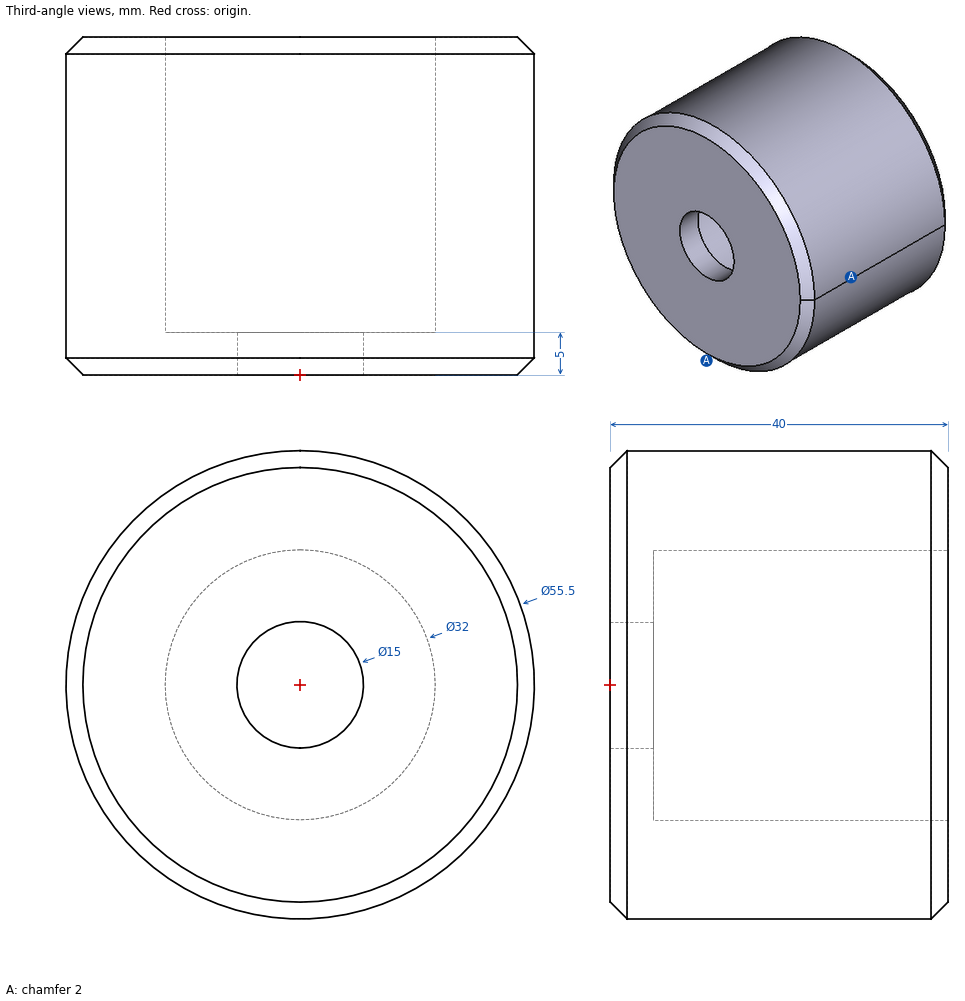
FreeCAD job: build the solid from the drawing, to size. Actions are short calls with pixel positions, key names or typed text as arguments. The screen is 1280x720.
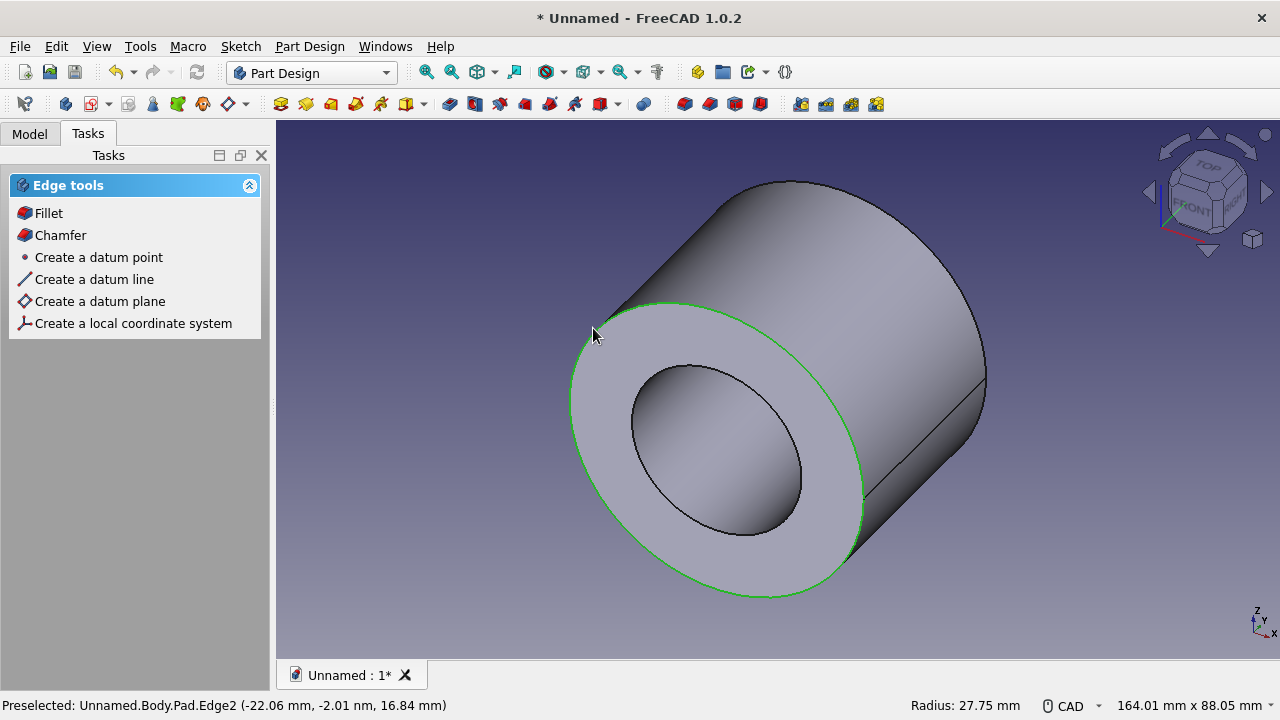
key(0)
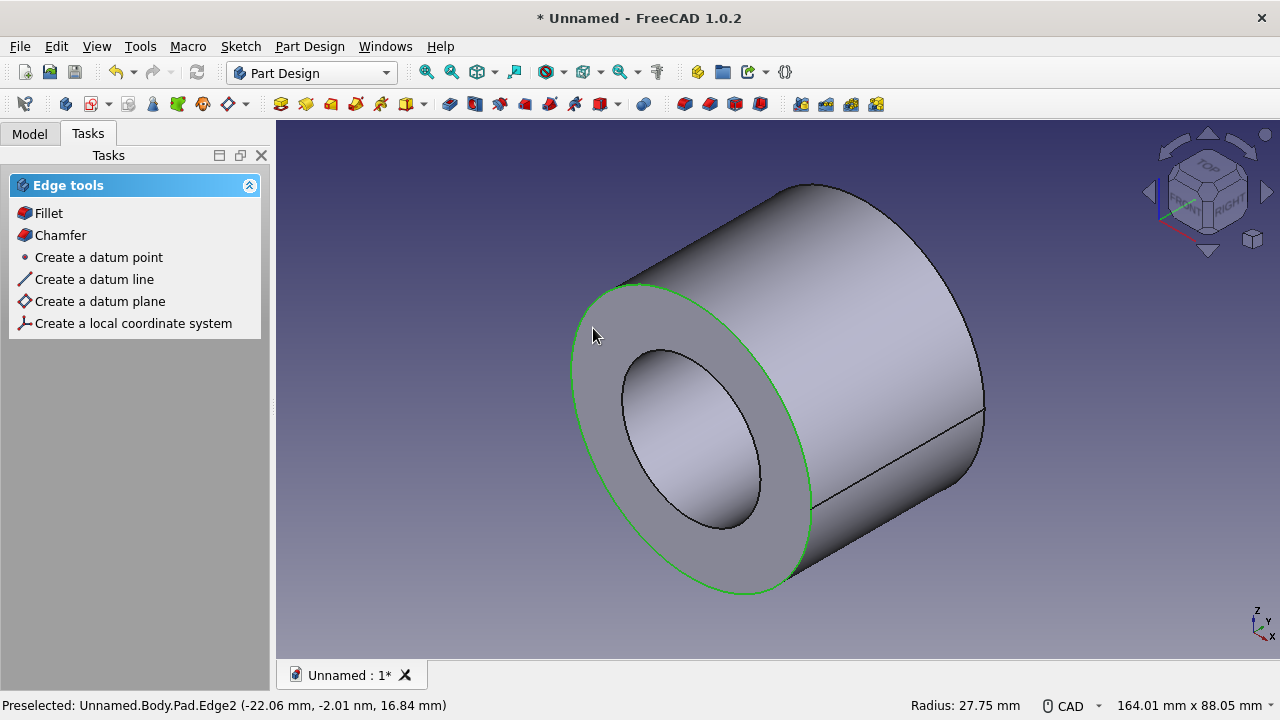
key(2)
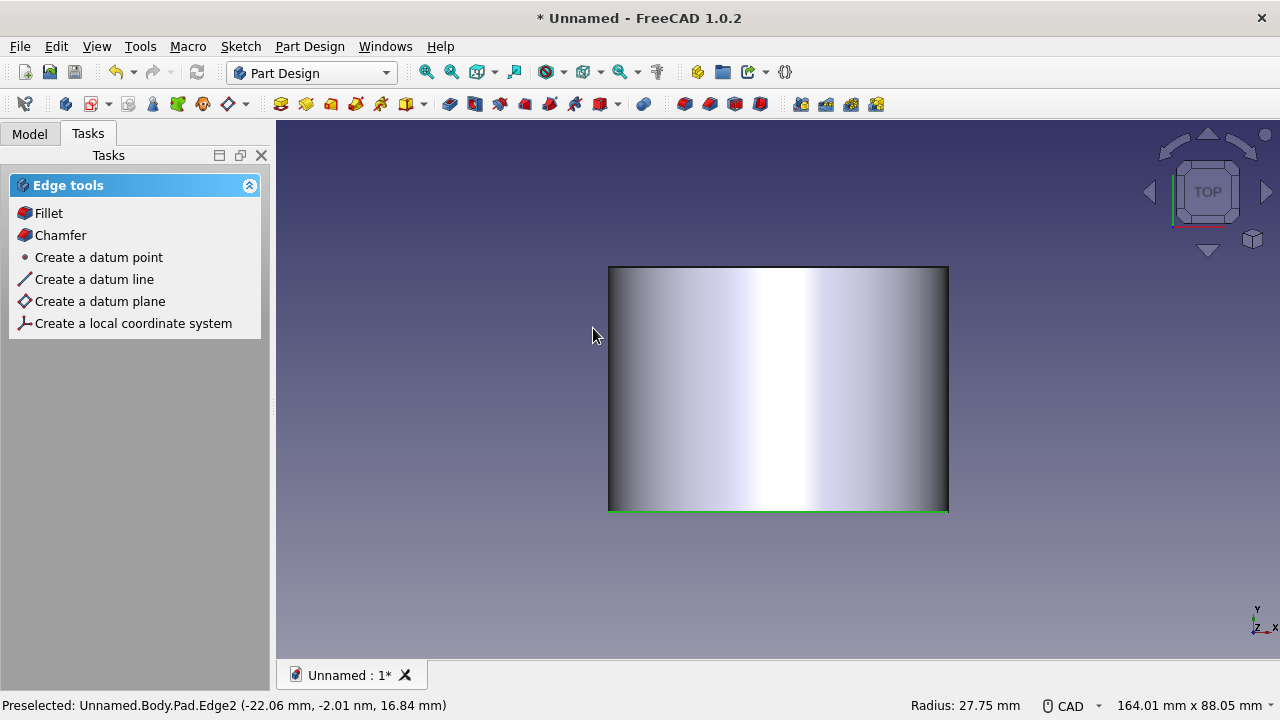
click(640, 266, ctrl)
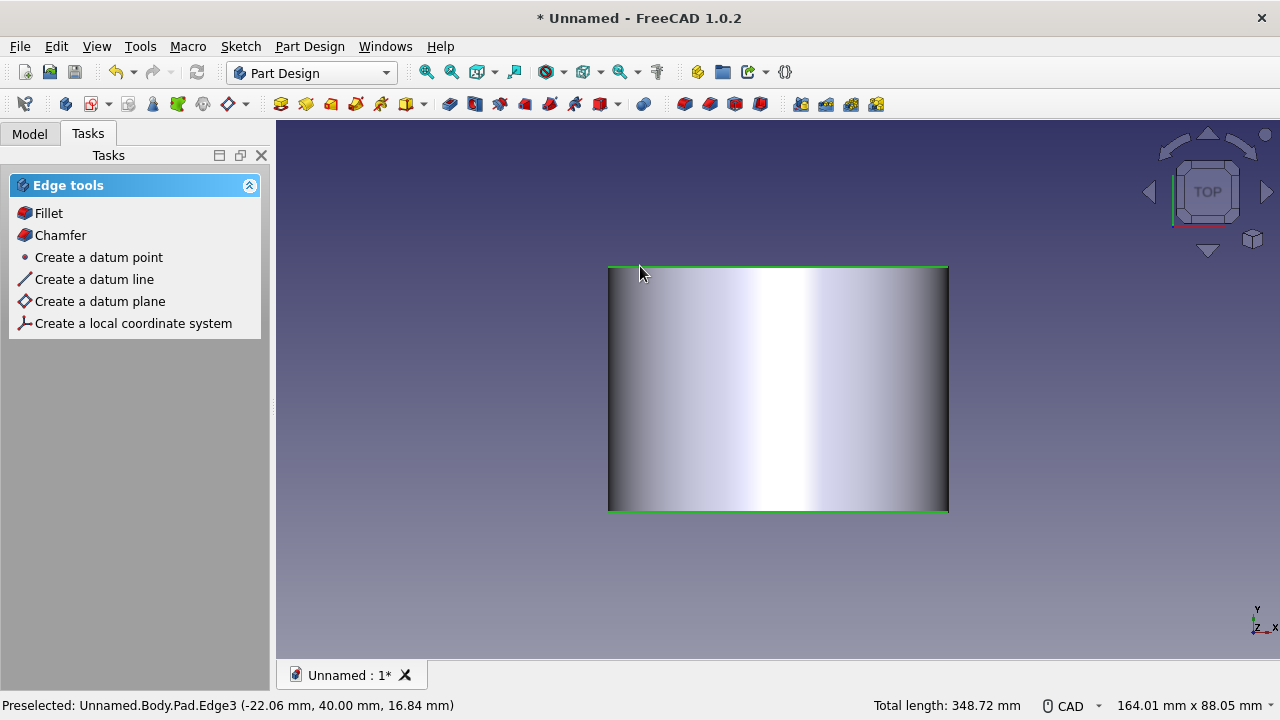
click(710, 104)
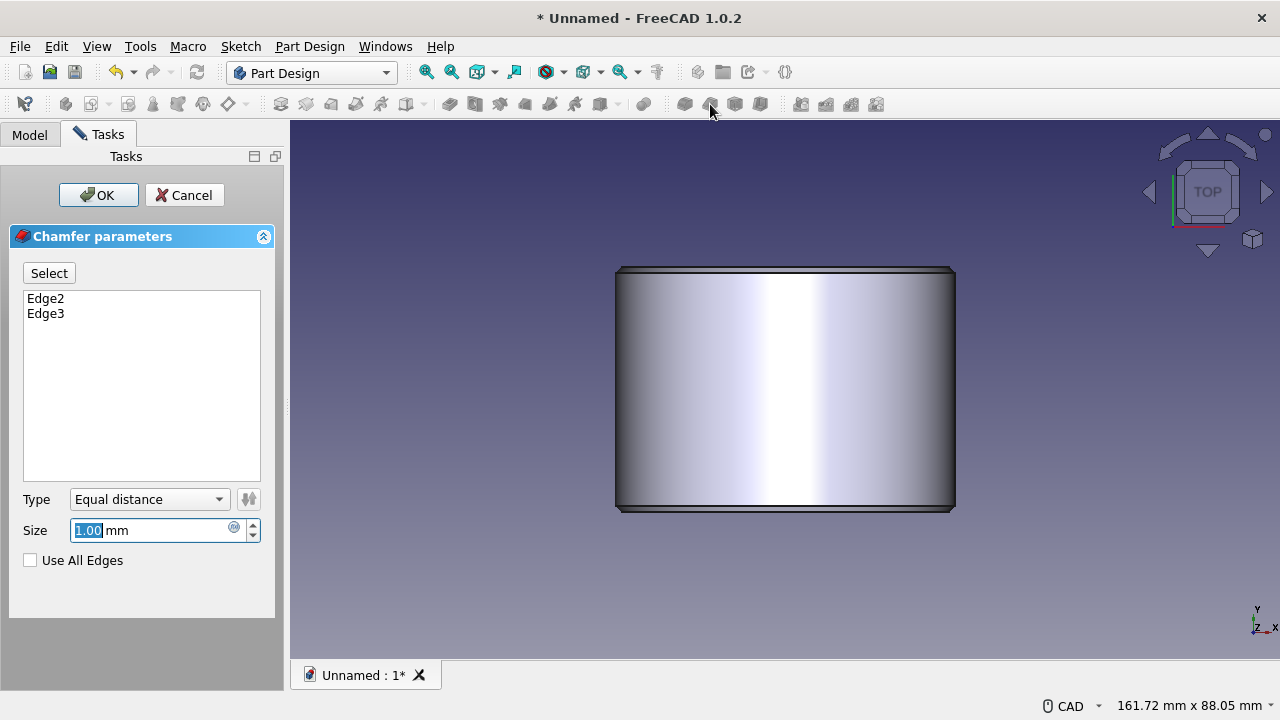
text(2)
key(Tab)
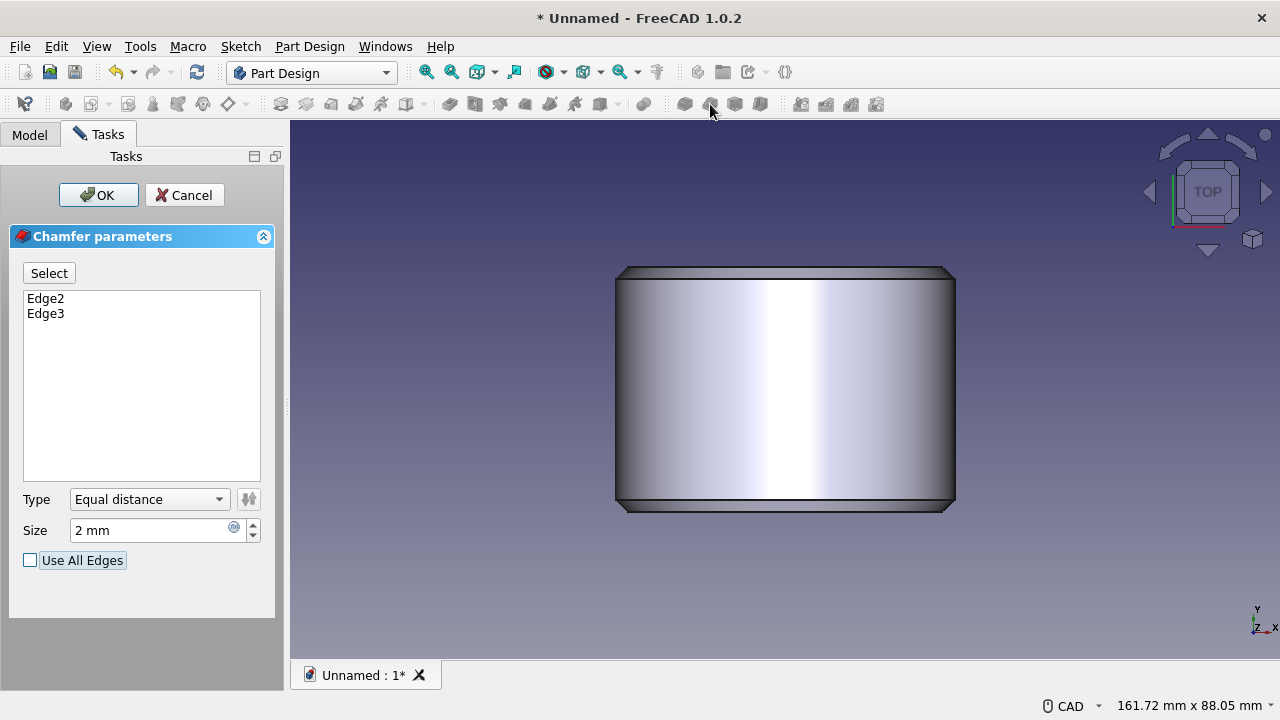
click(99, 195)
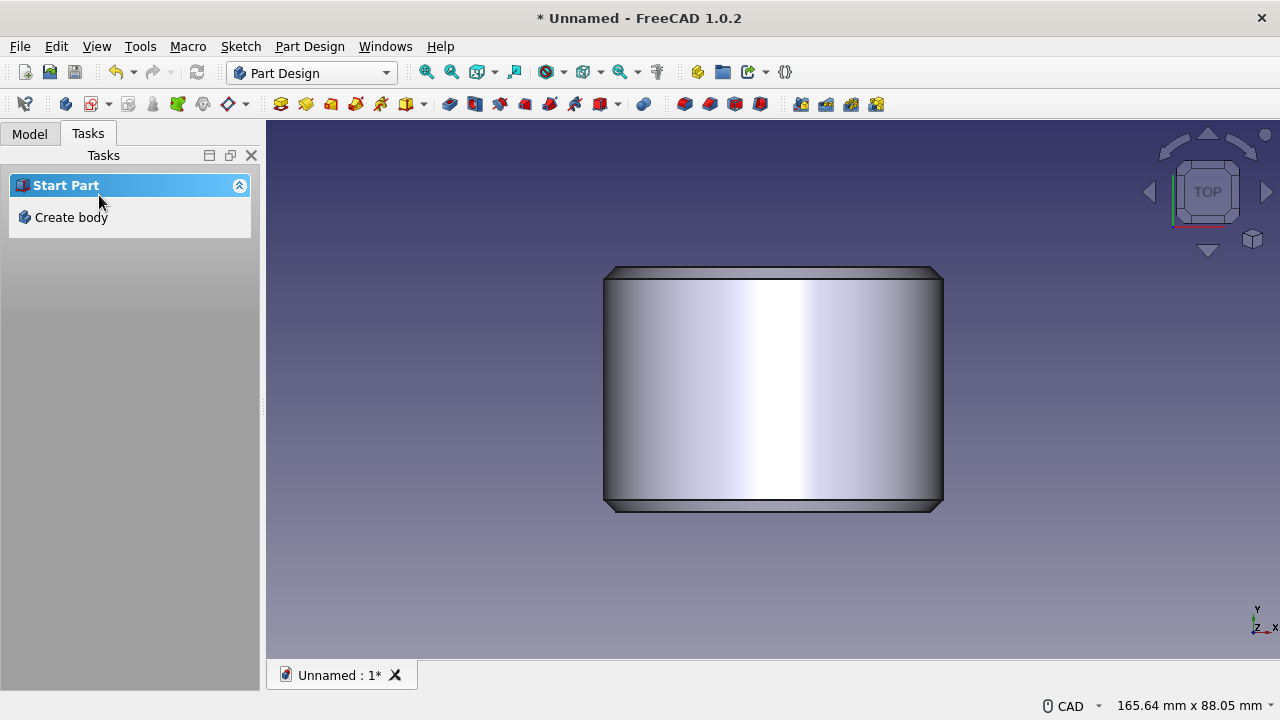
key(0)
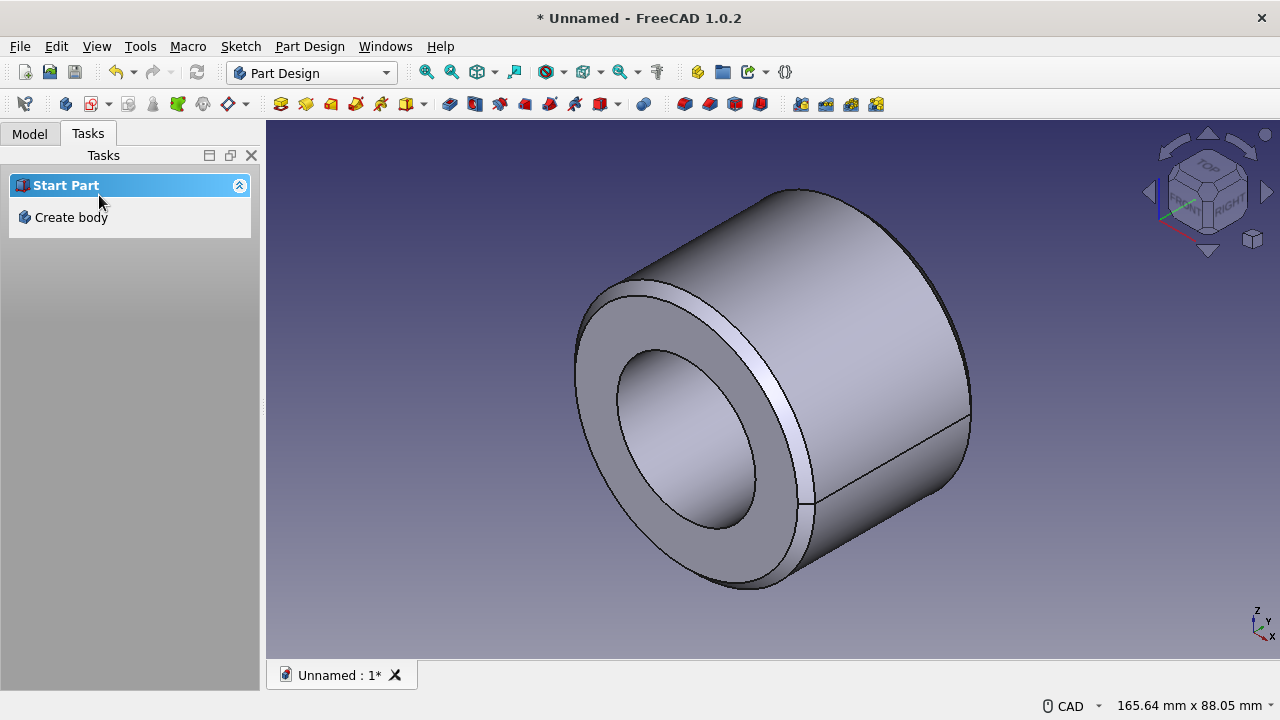
click(750, 402)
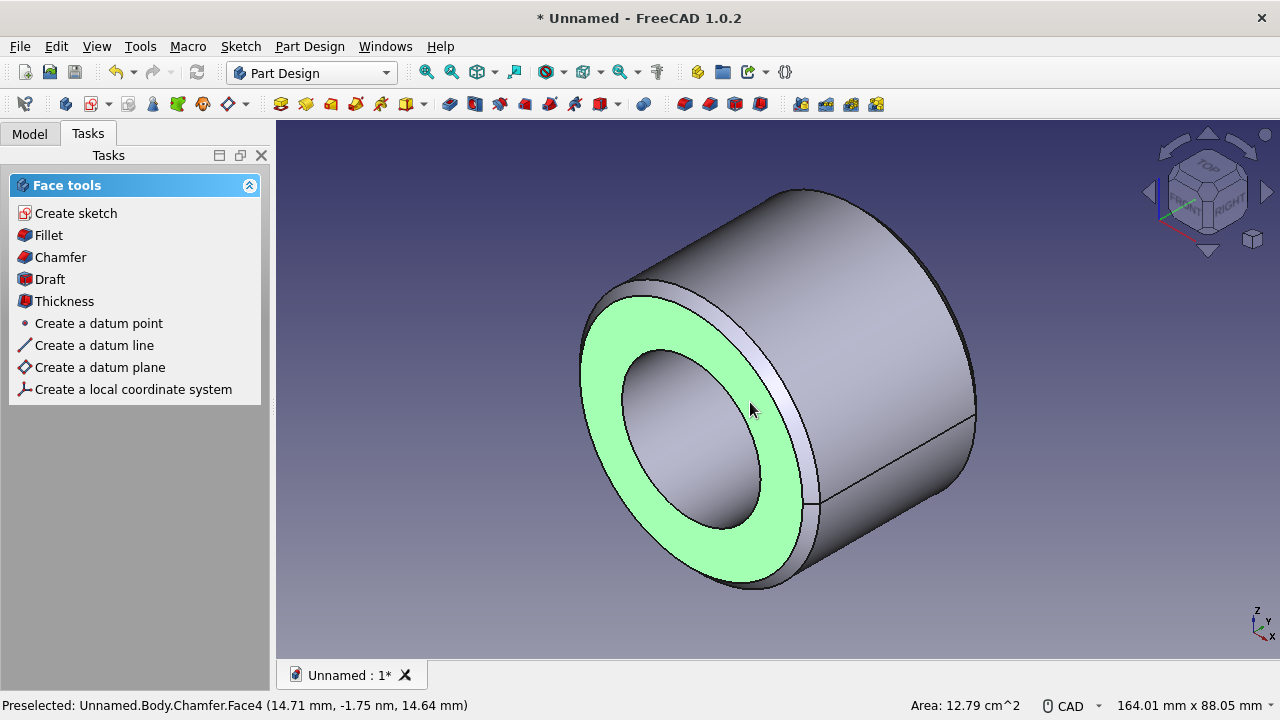
click(90, 104)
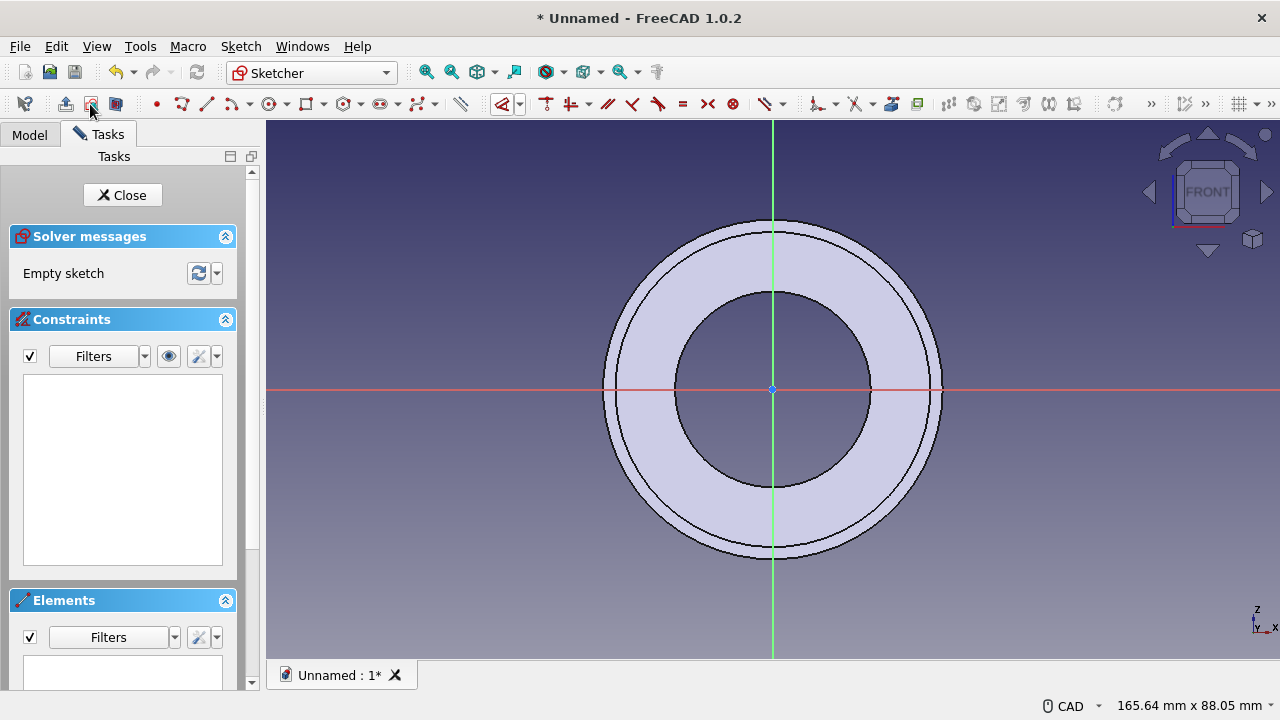
scroll(856, 390, up, 3)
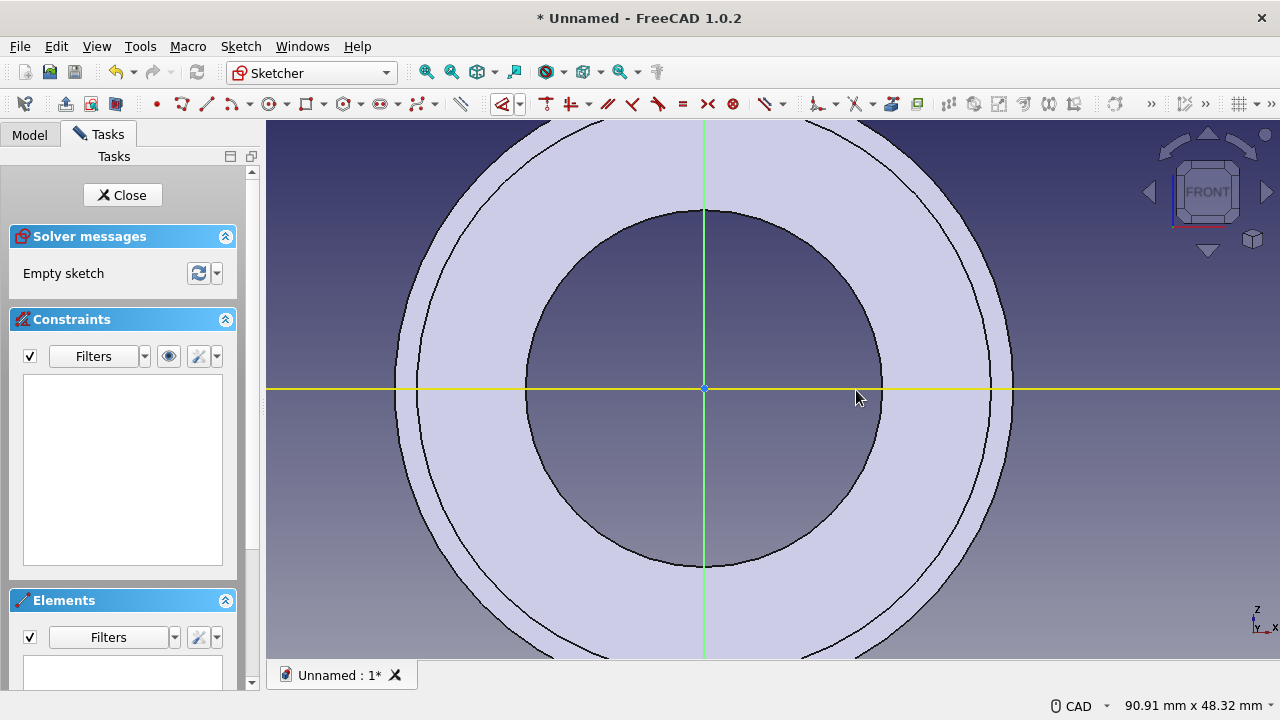
click(268, 104)